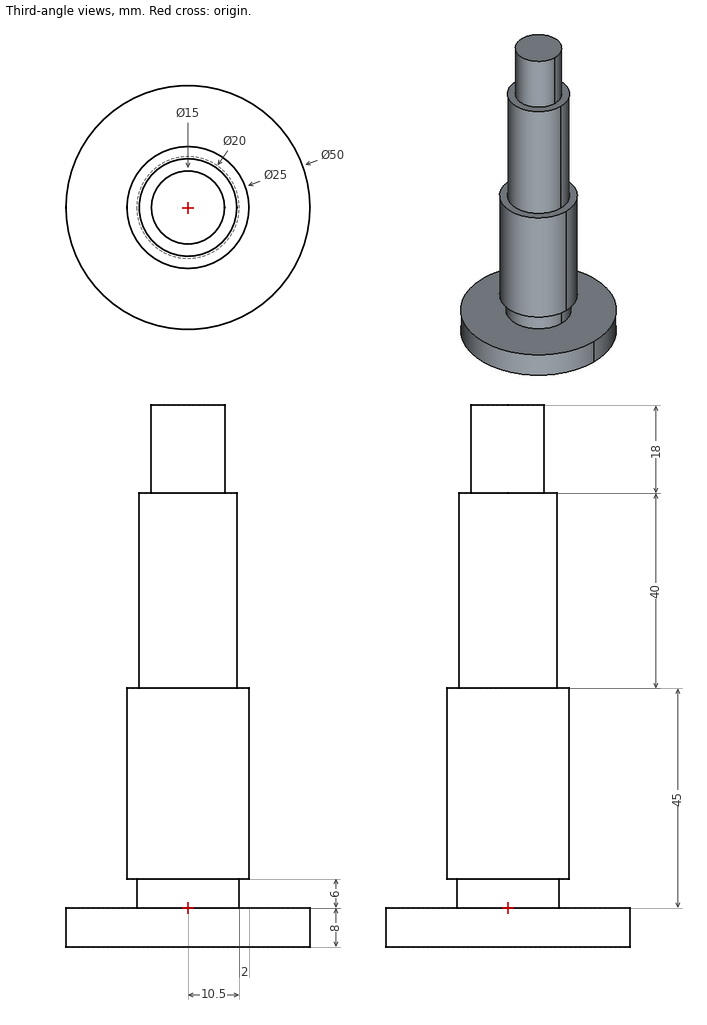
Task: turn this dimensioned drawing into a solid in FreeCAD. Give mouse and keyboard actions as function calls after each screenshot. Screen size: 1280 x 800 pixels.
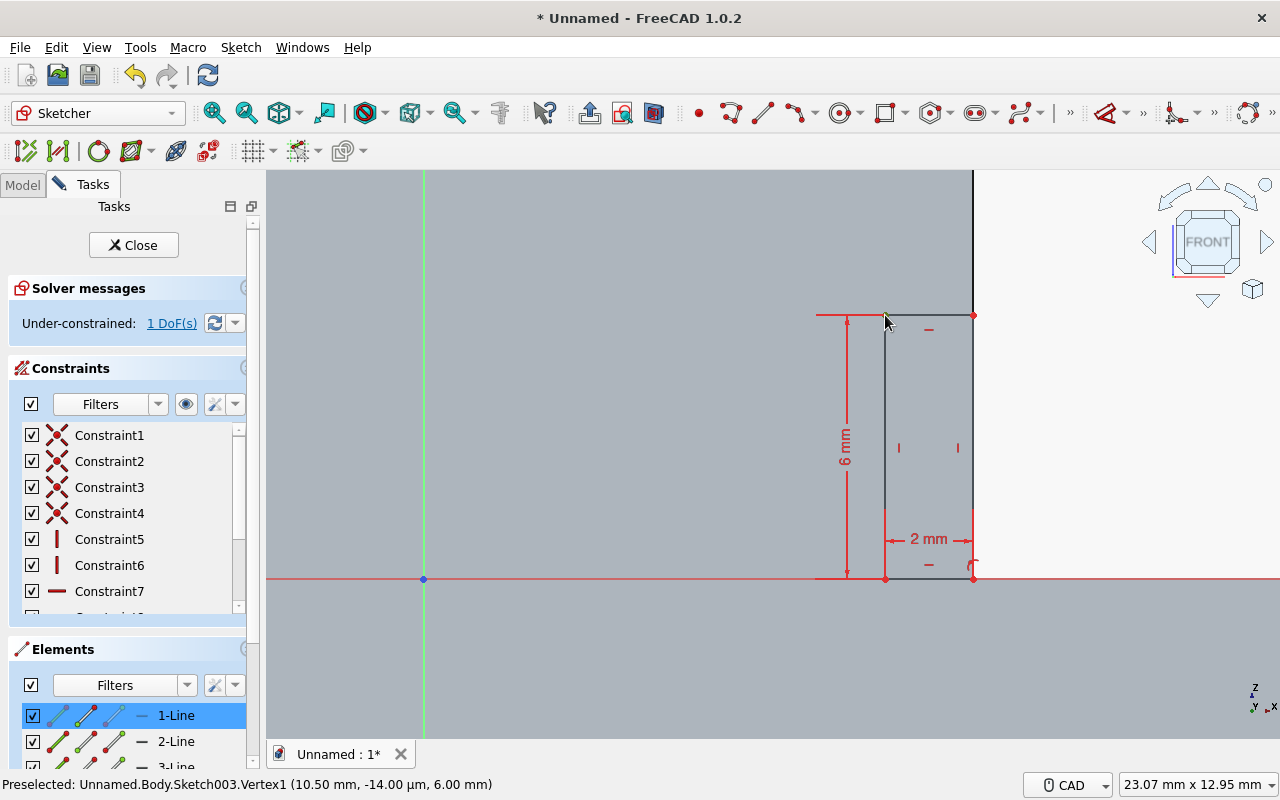
key(l)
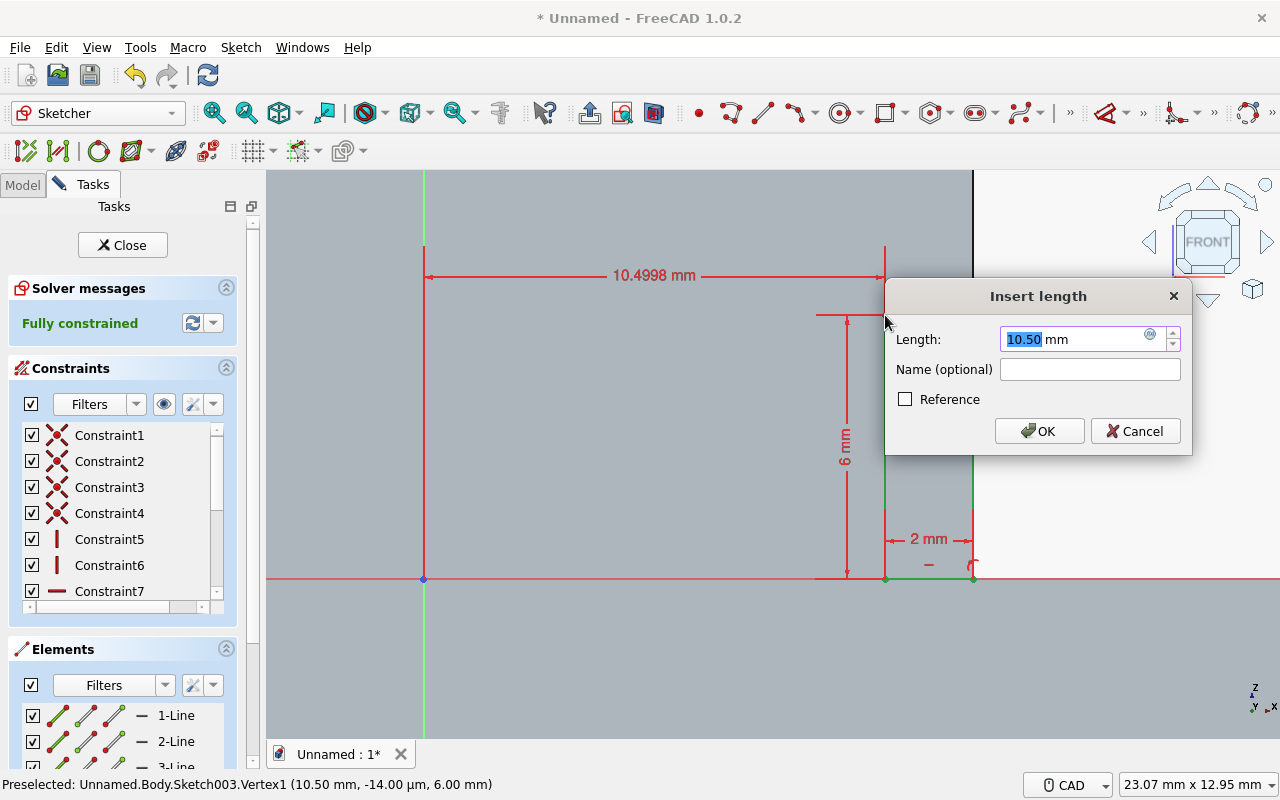
text(10.5)
key(Return)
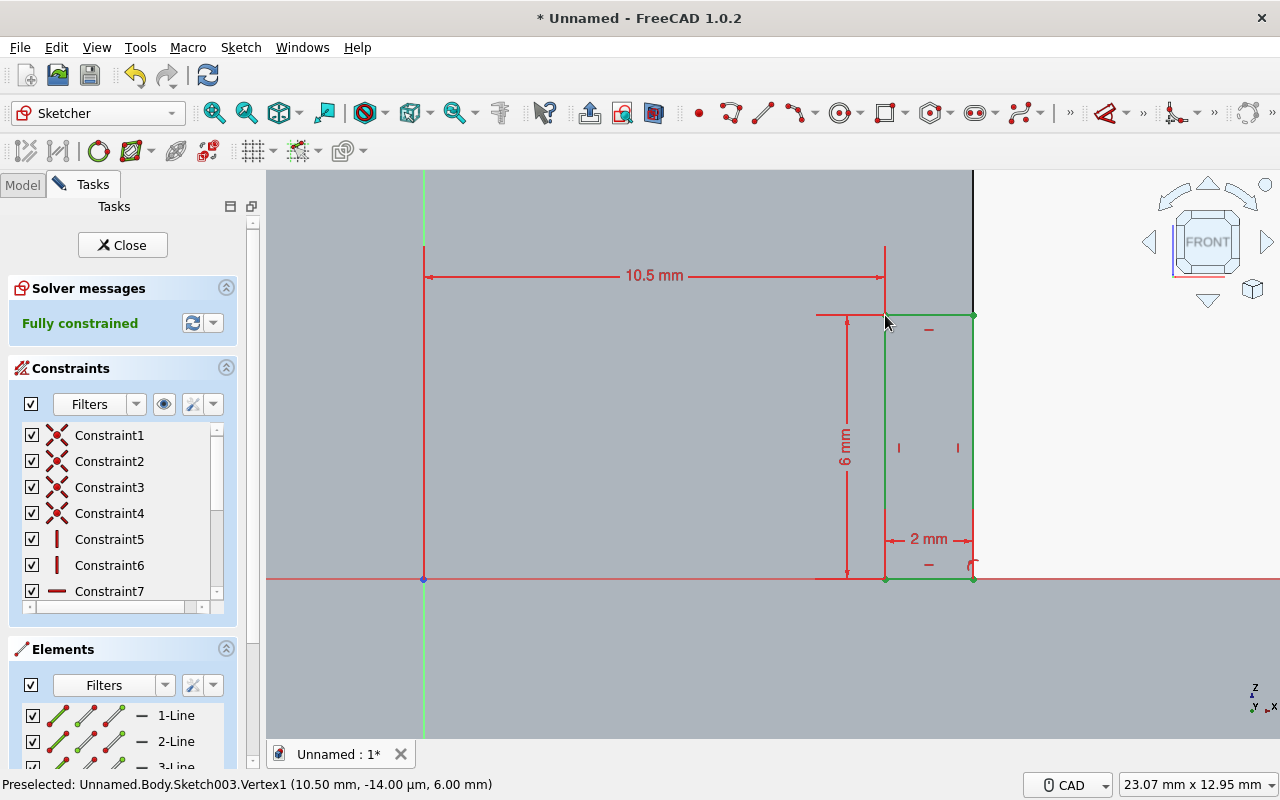
click(123, 245)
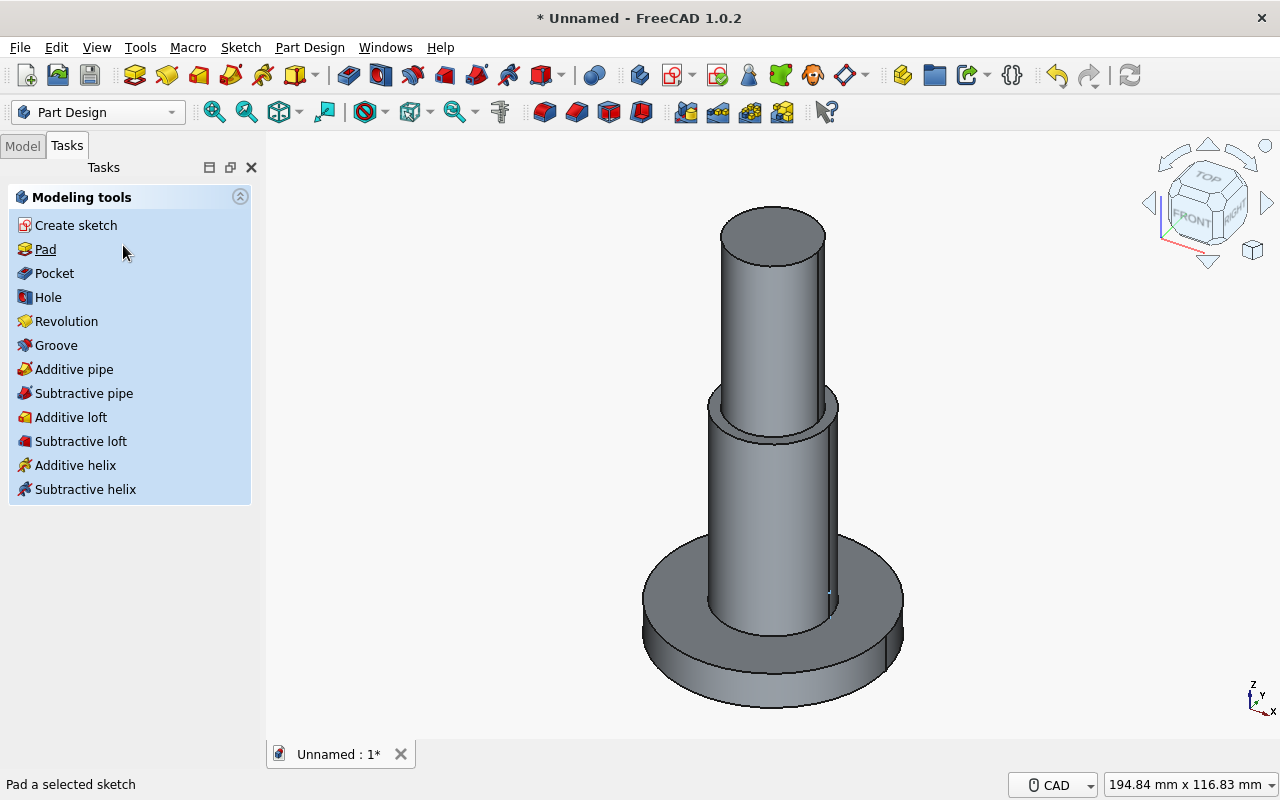
click(414, 76)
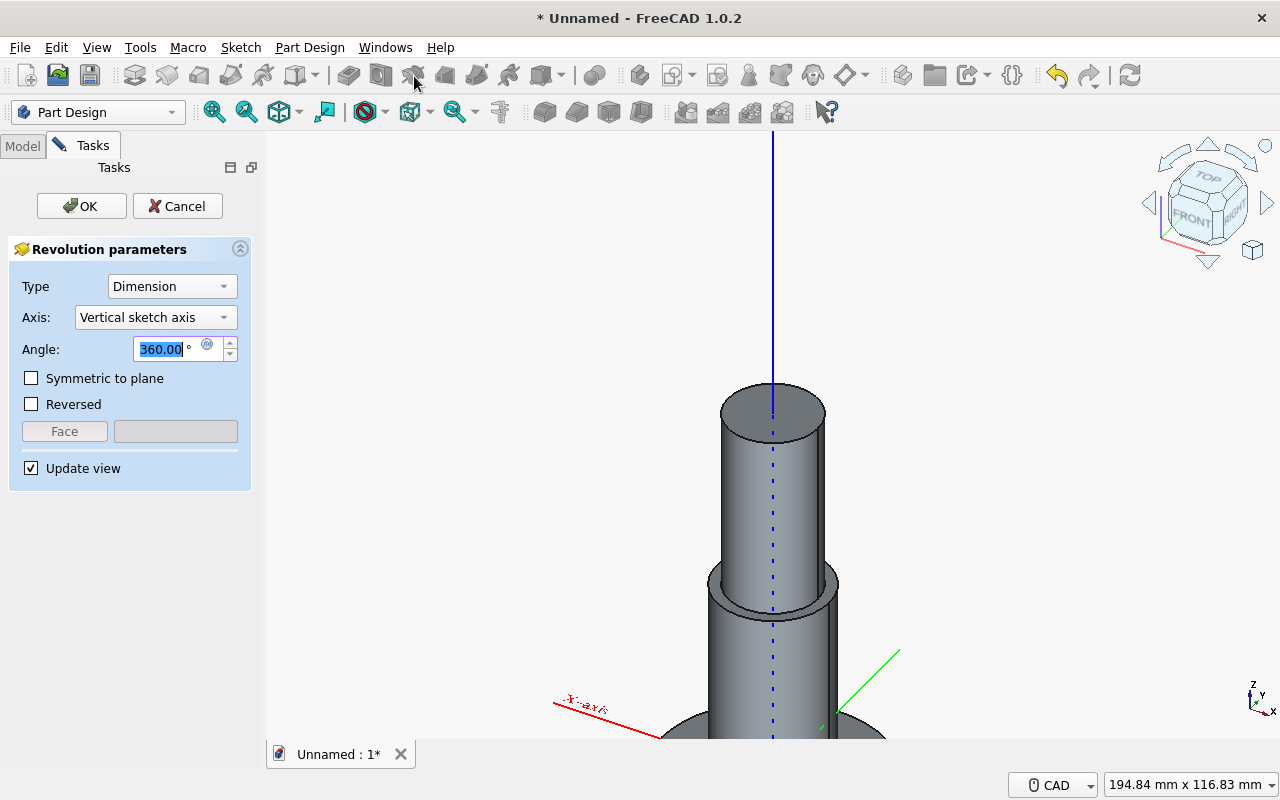
click(82, 206)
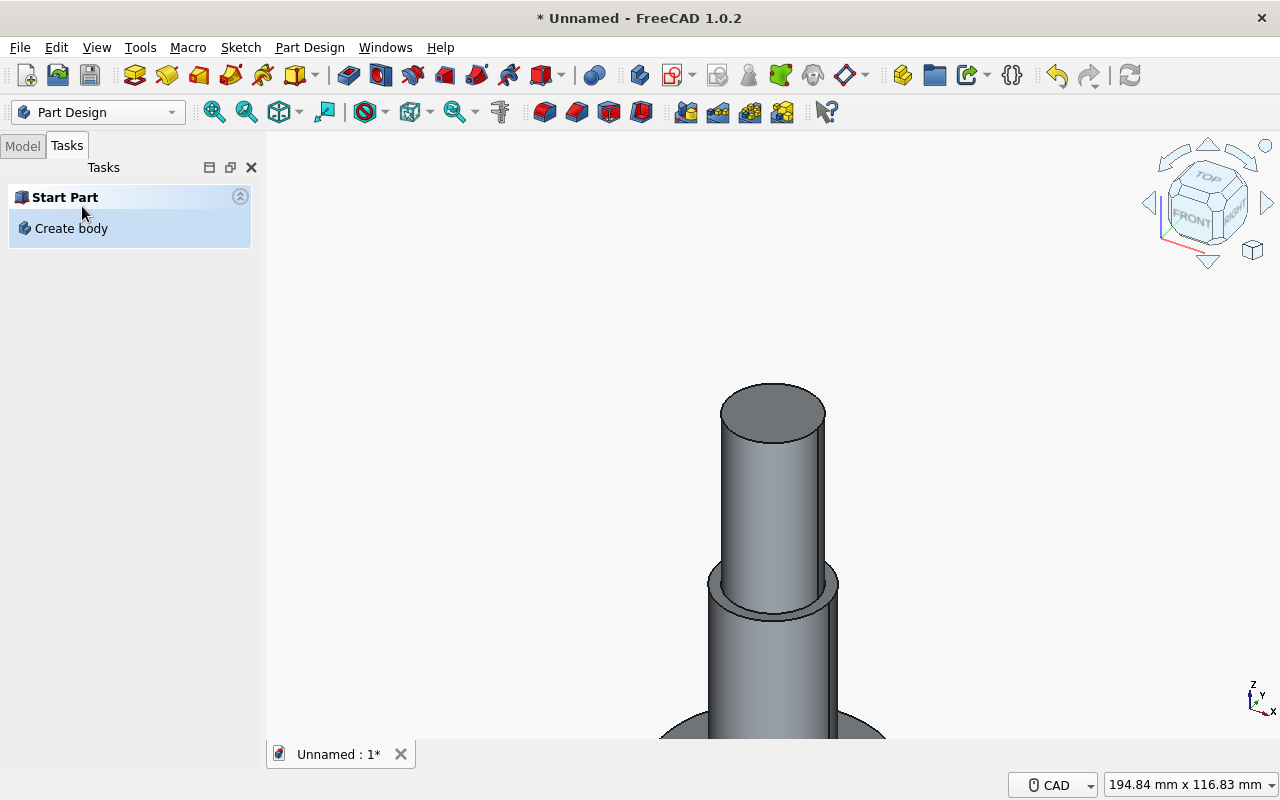
key(v)
key(f)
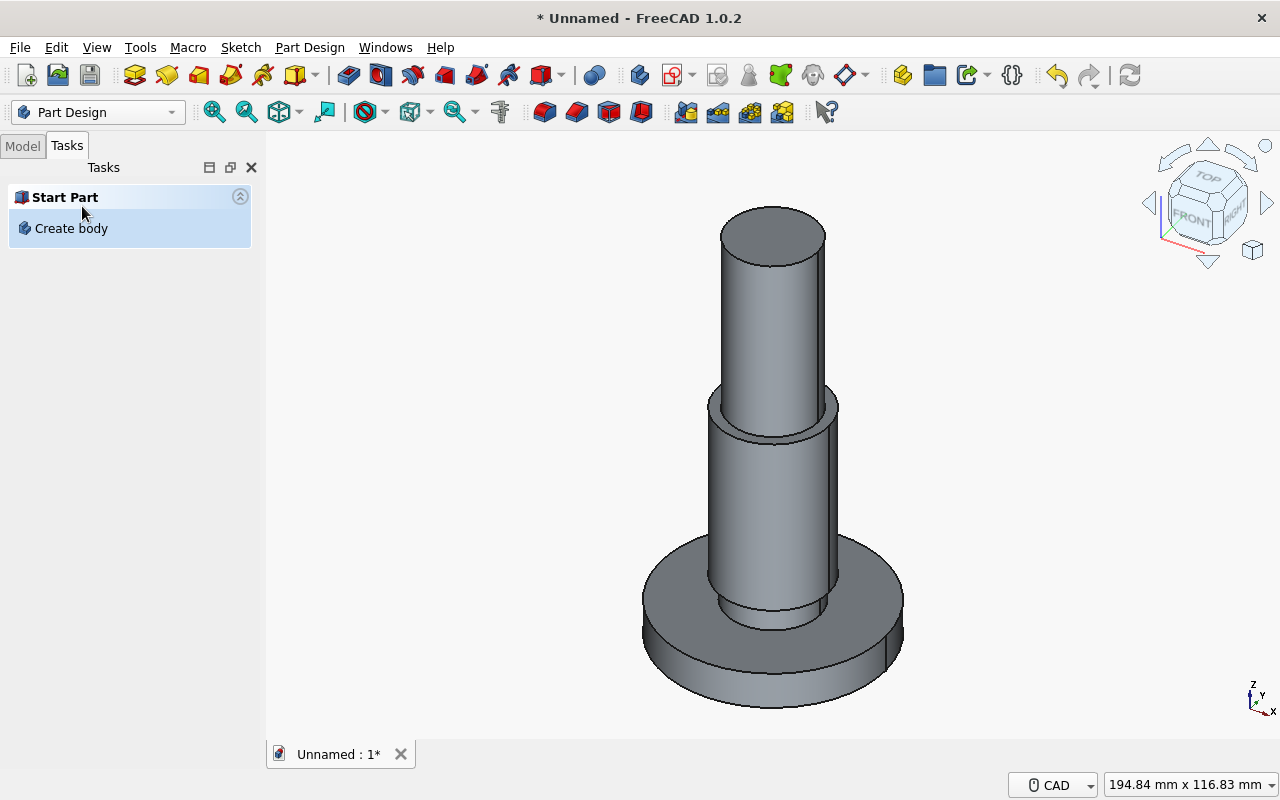
click(773, 236)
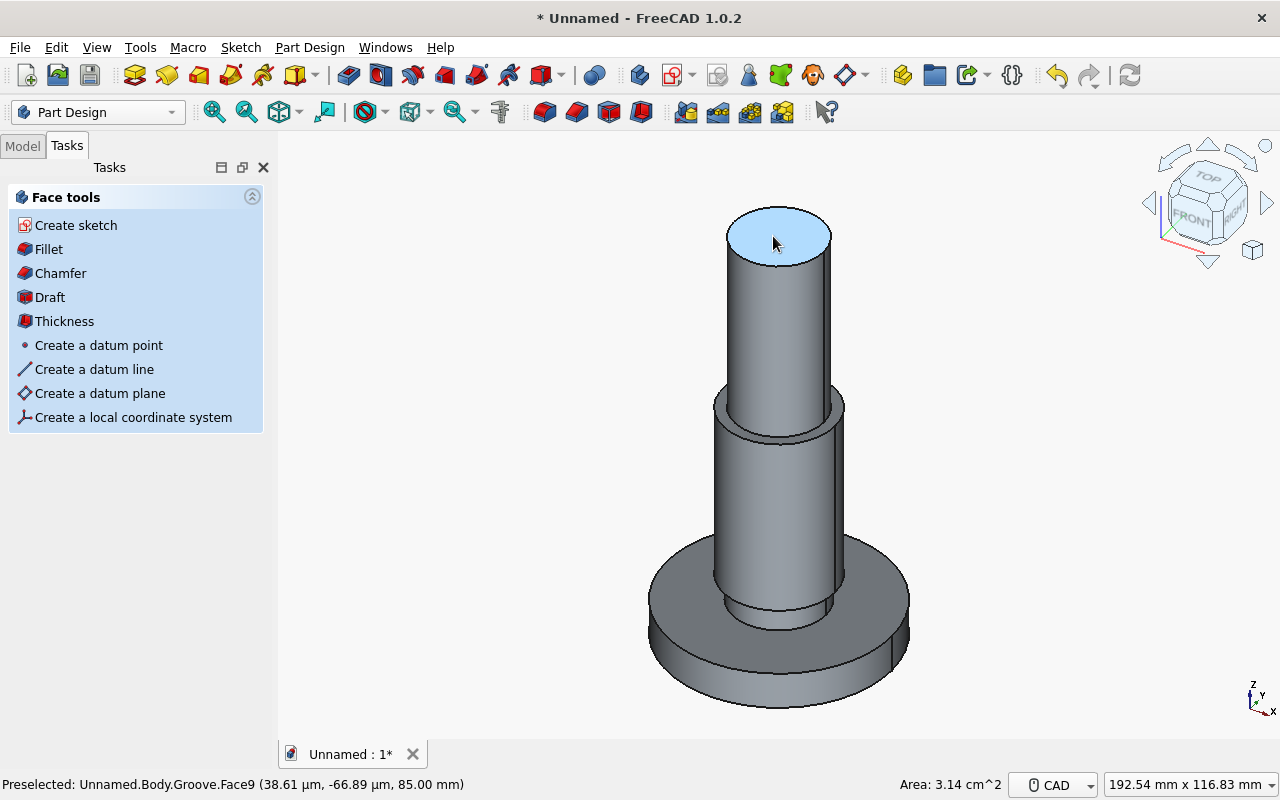
click(672, 76)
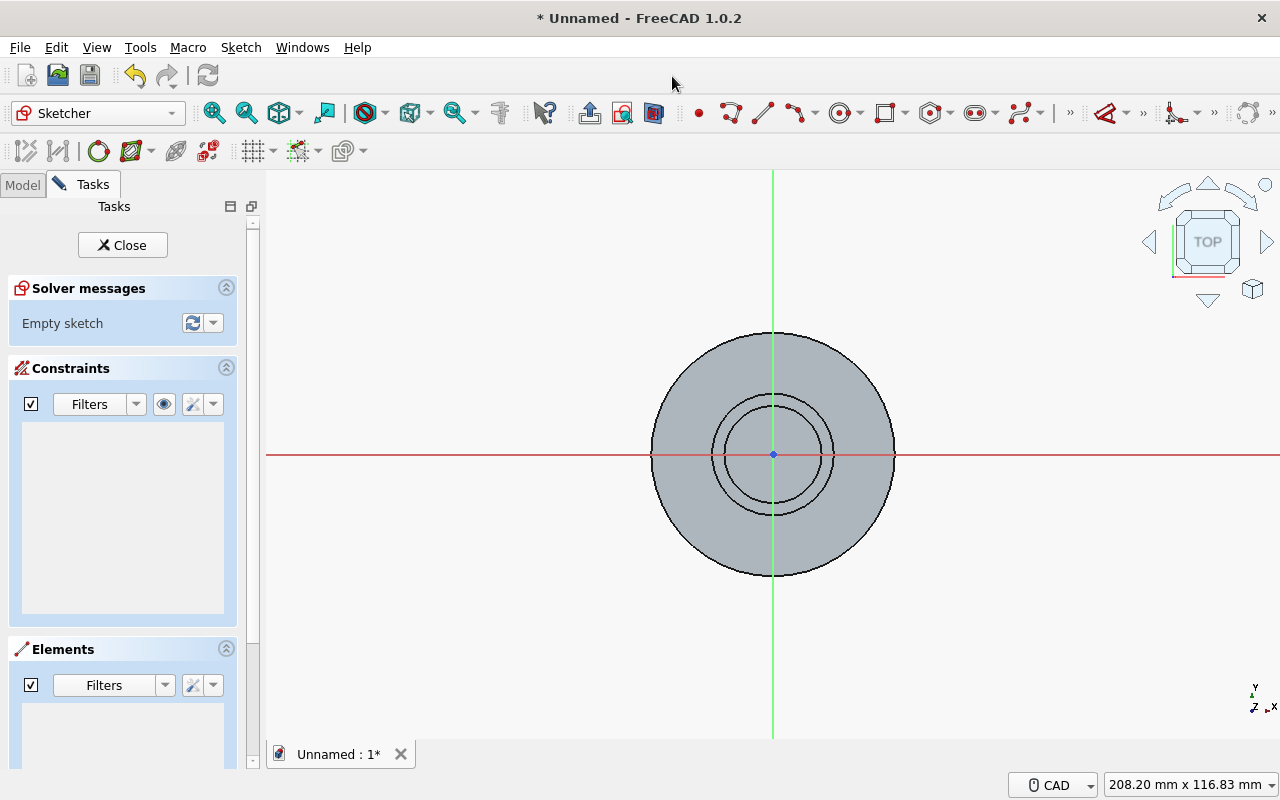
scroll(790, 454, up, 8)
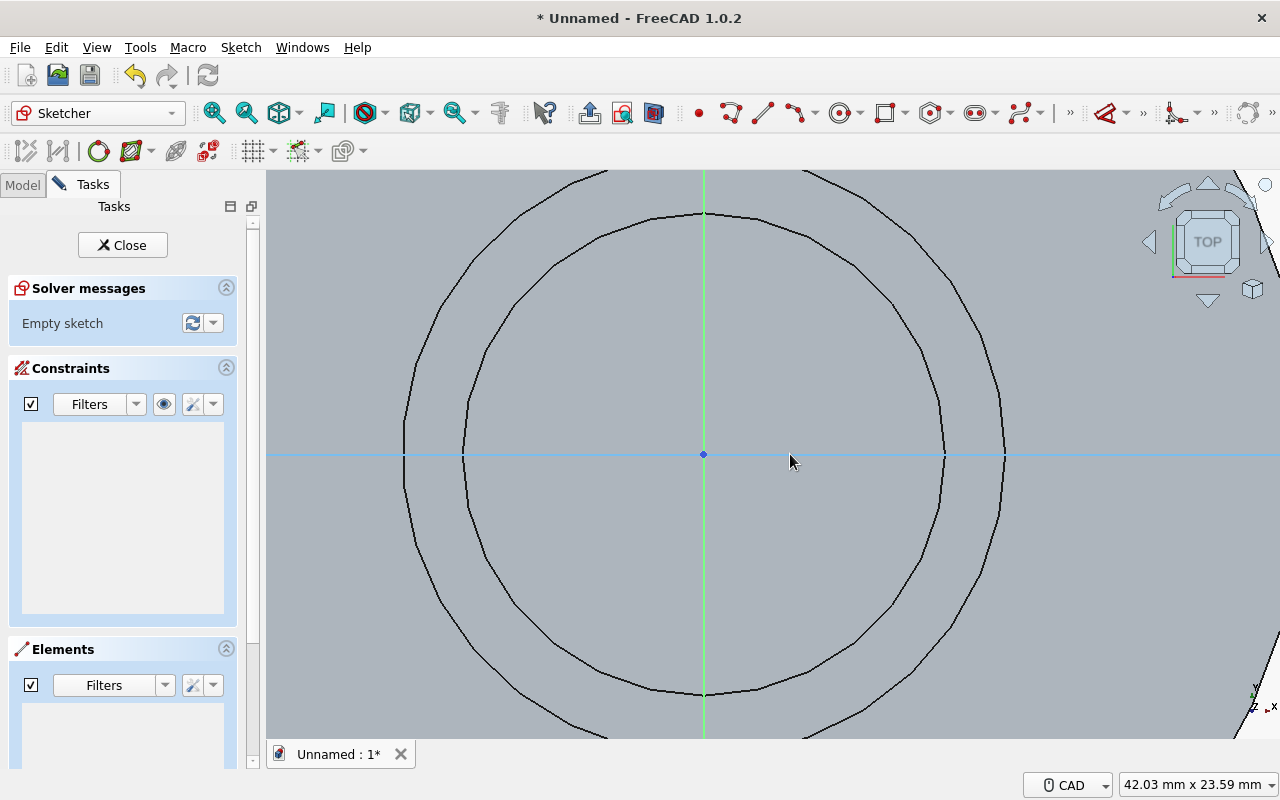
click(840, 114)